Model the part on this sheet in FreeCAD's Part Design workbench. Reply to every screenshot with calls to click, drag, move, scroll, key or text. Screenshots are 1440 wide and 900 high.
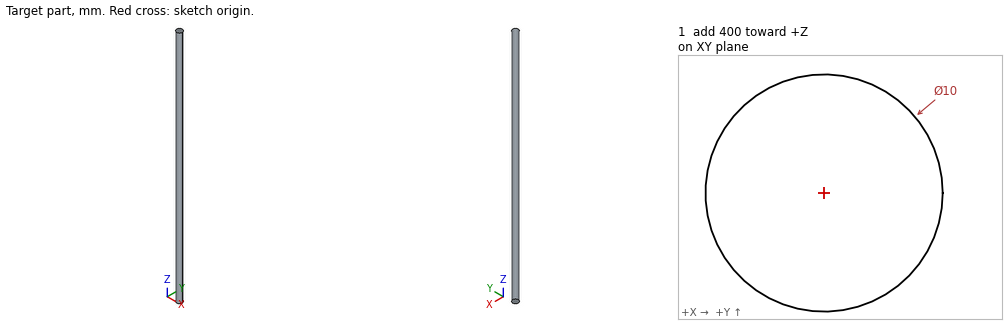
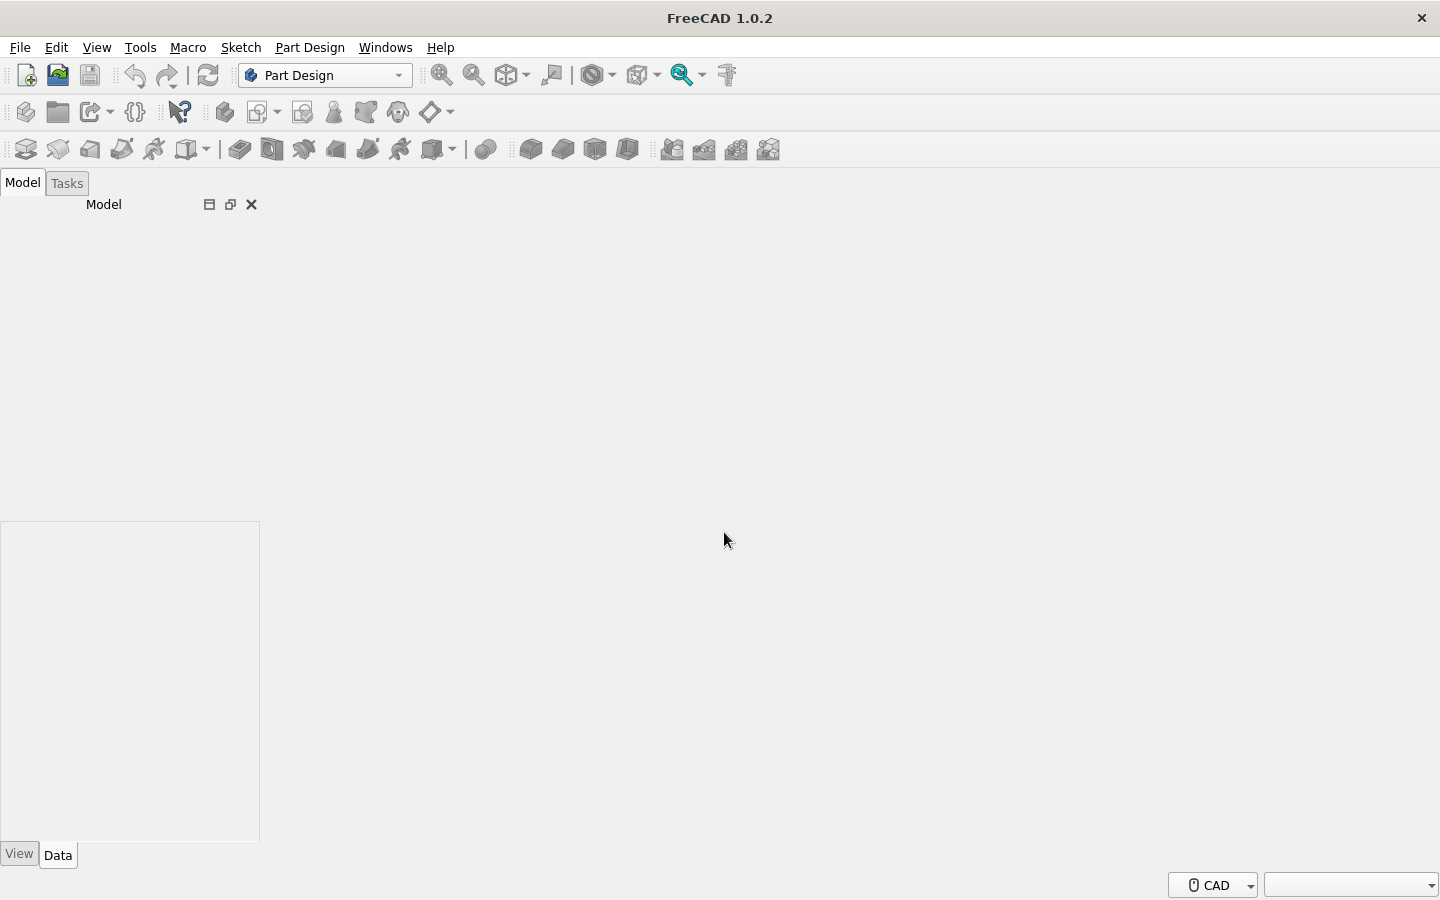
click(26, 76)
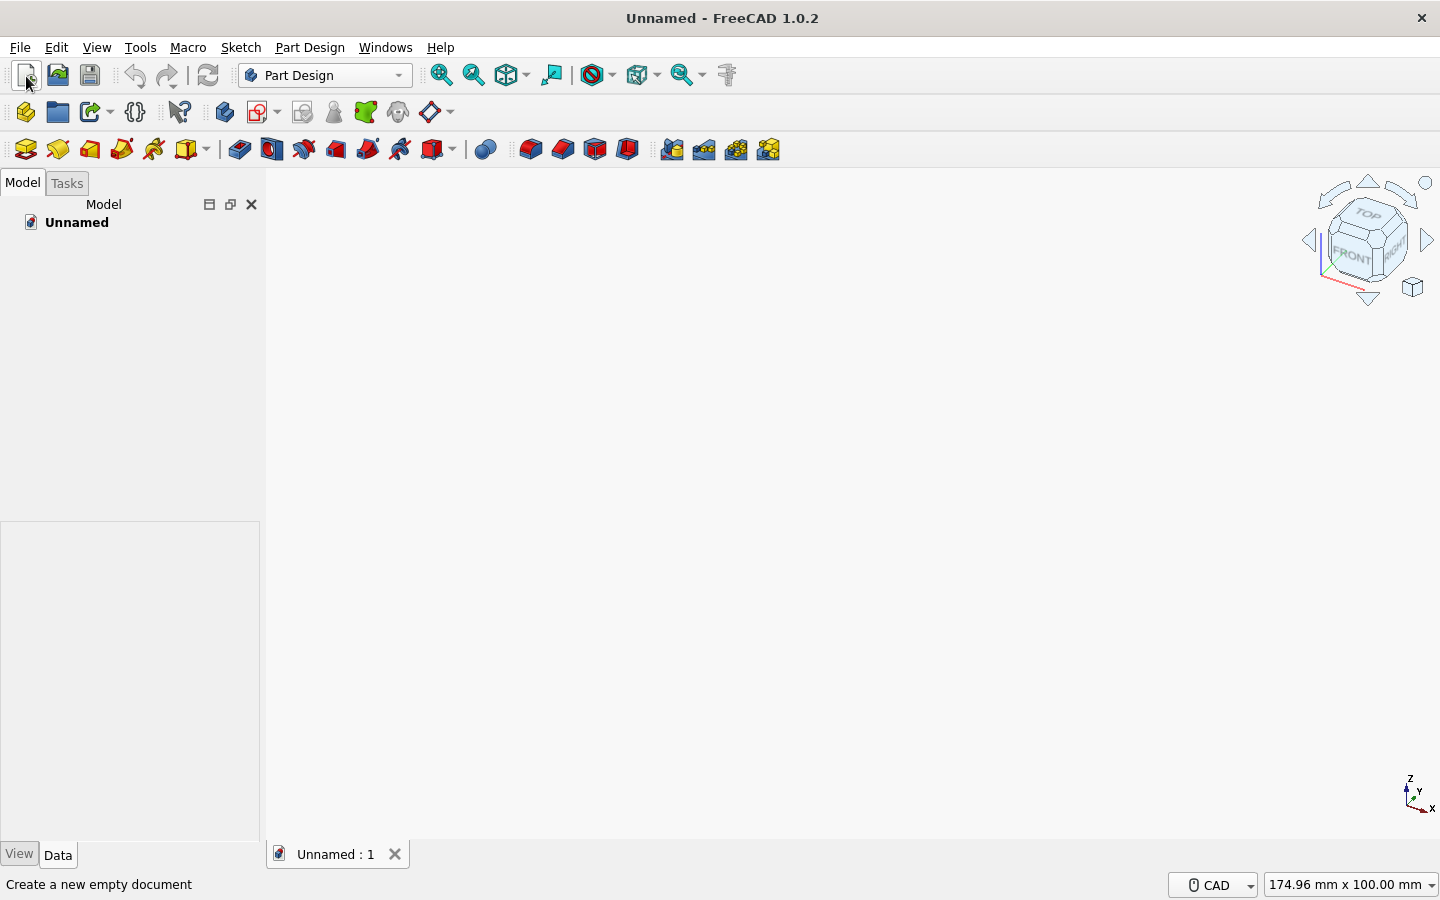
click(258, 112)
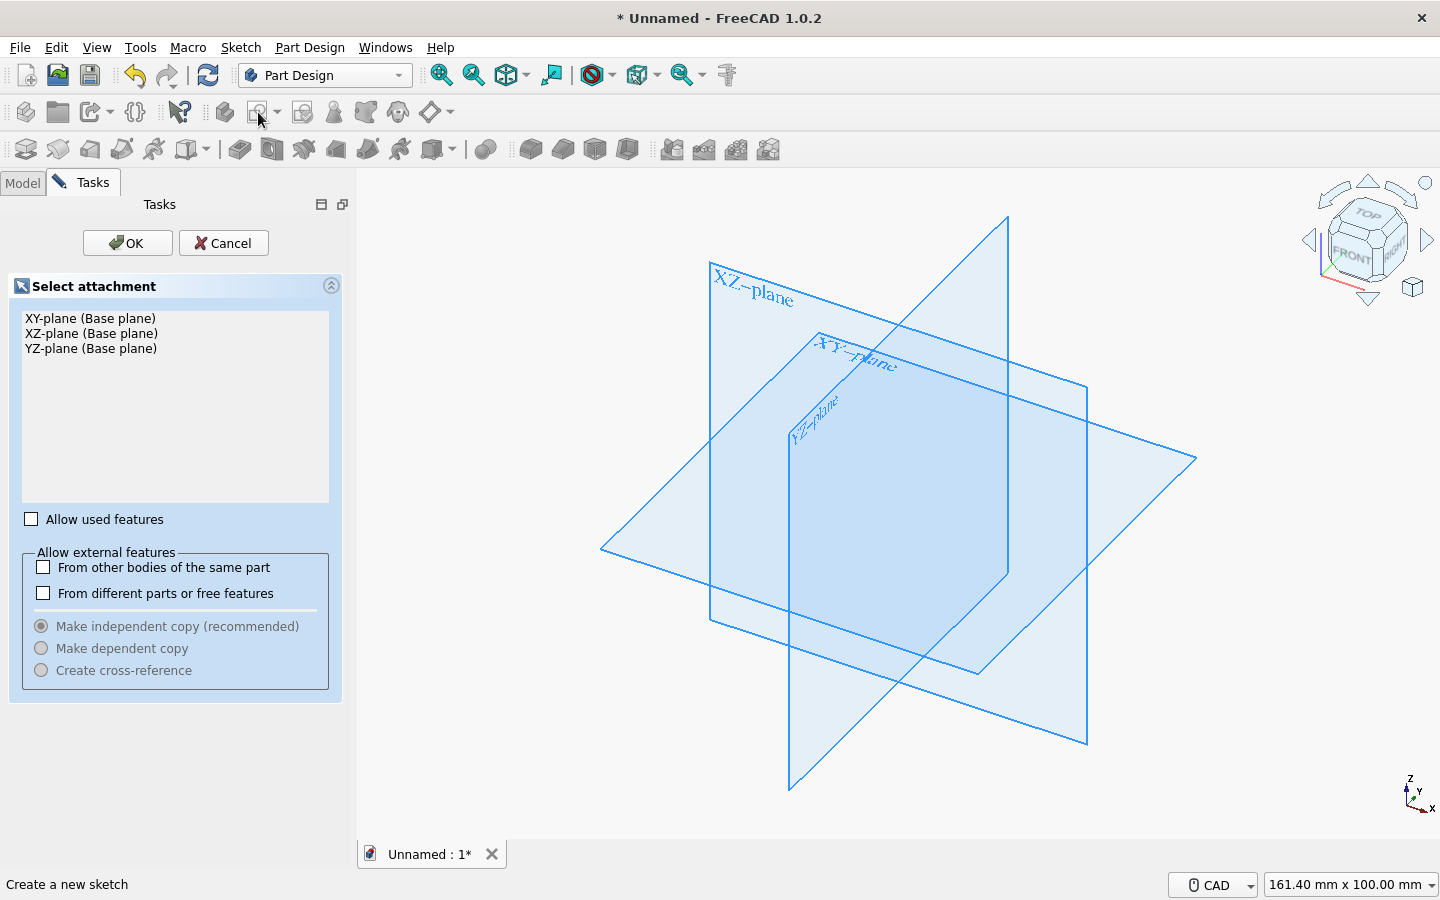
click(82, 318)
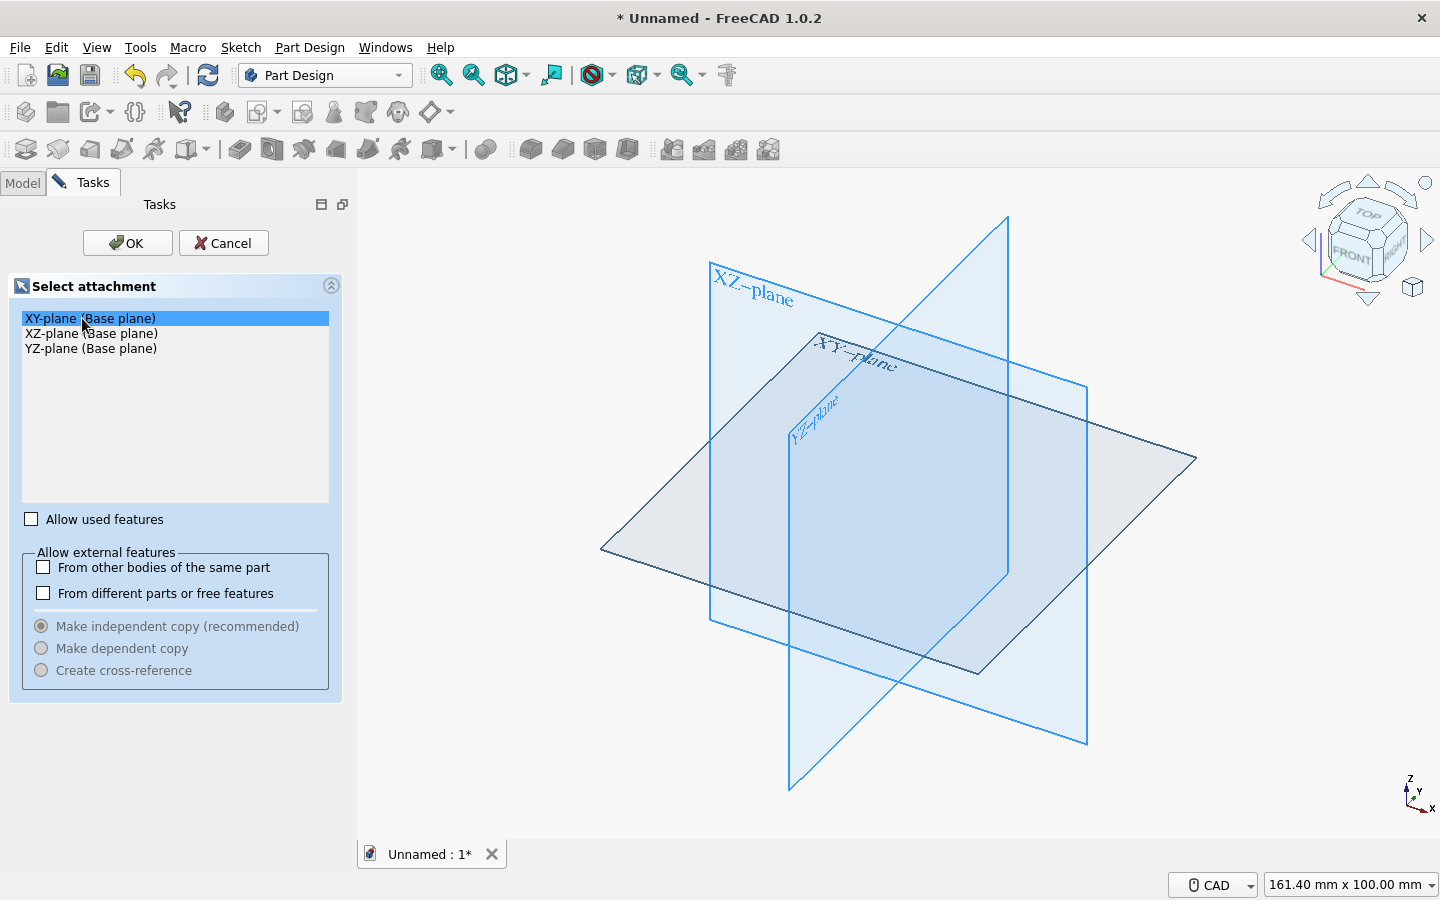
click(128, 243)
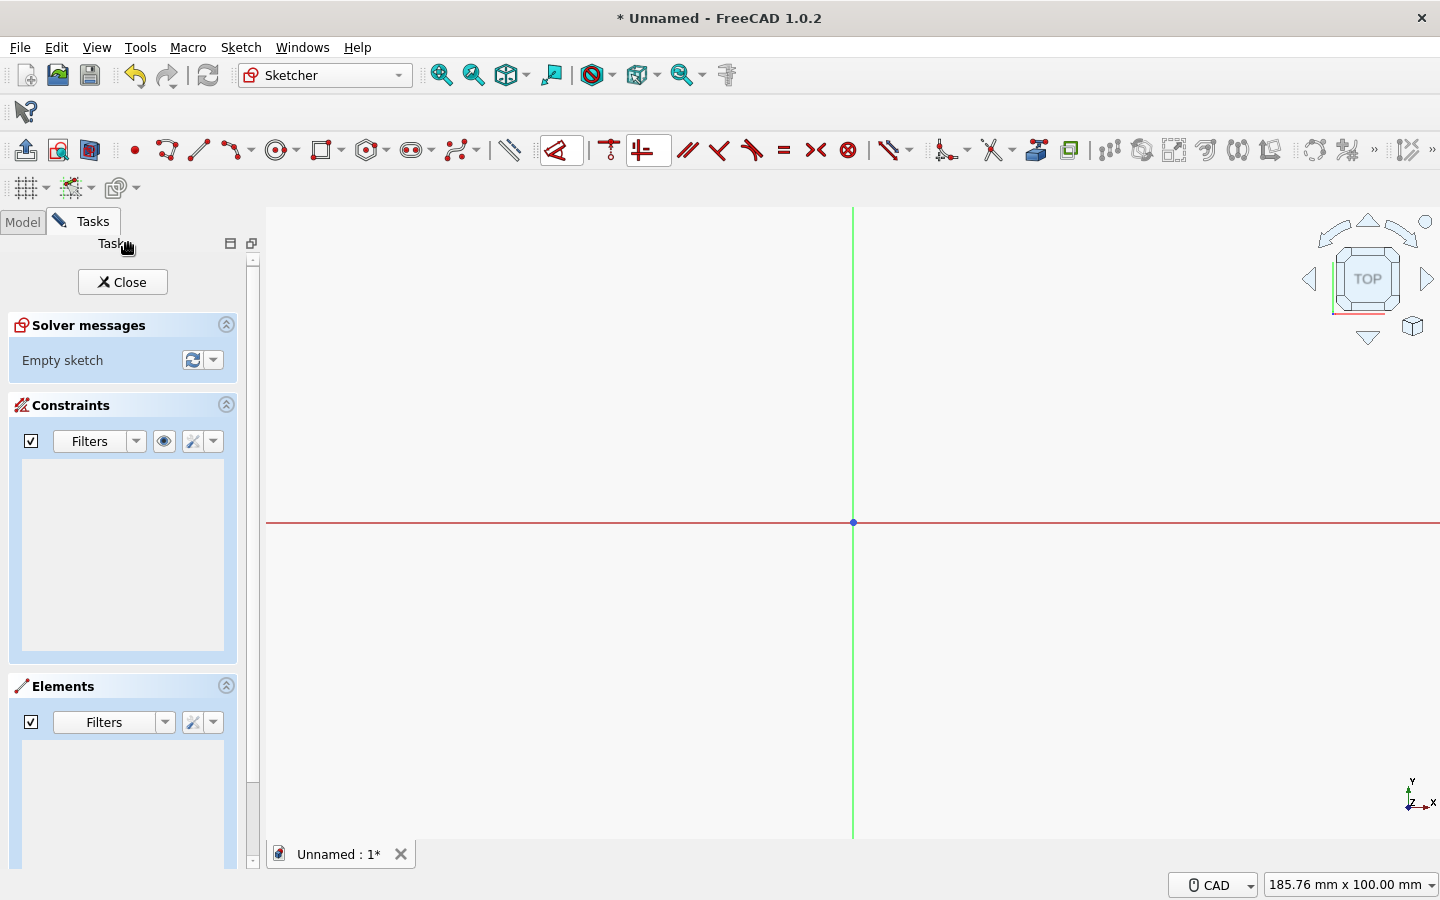
scroll(867, 523, up, 9)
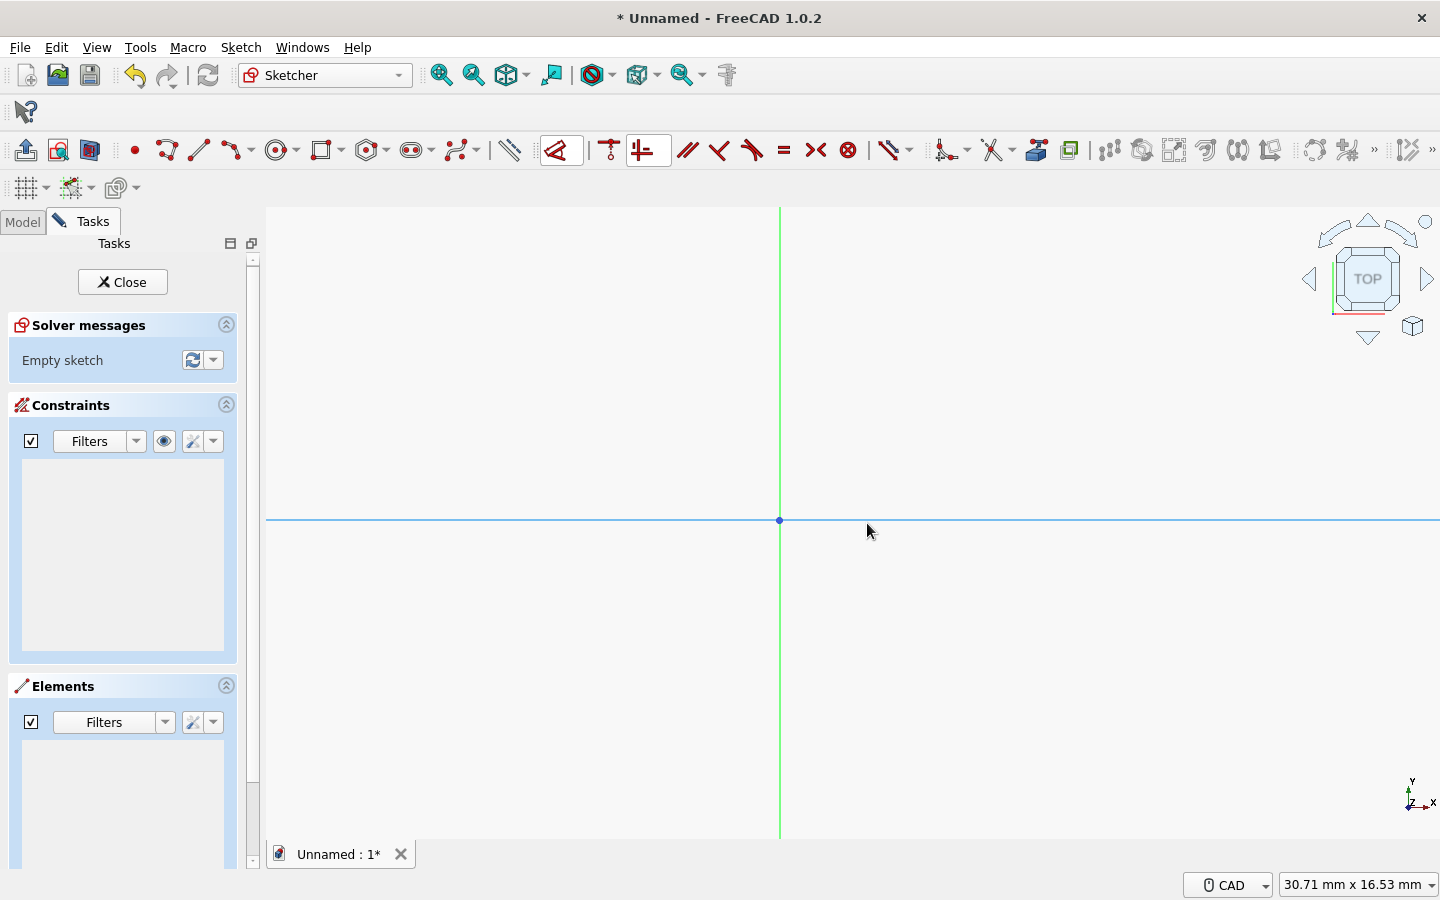
click(276, 150)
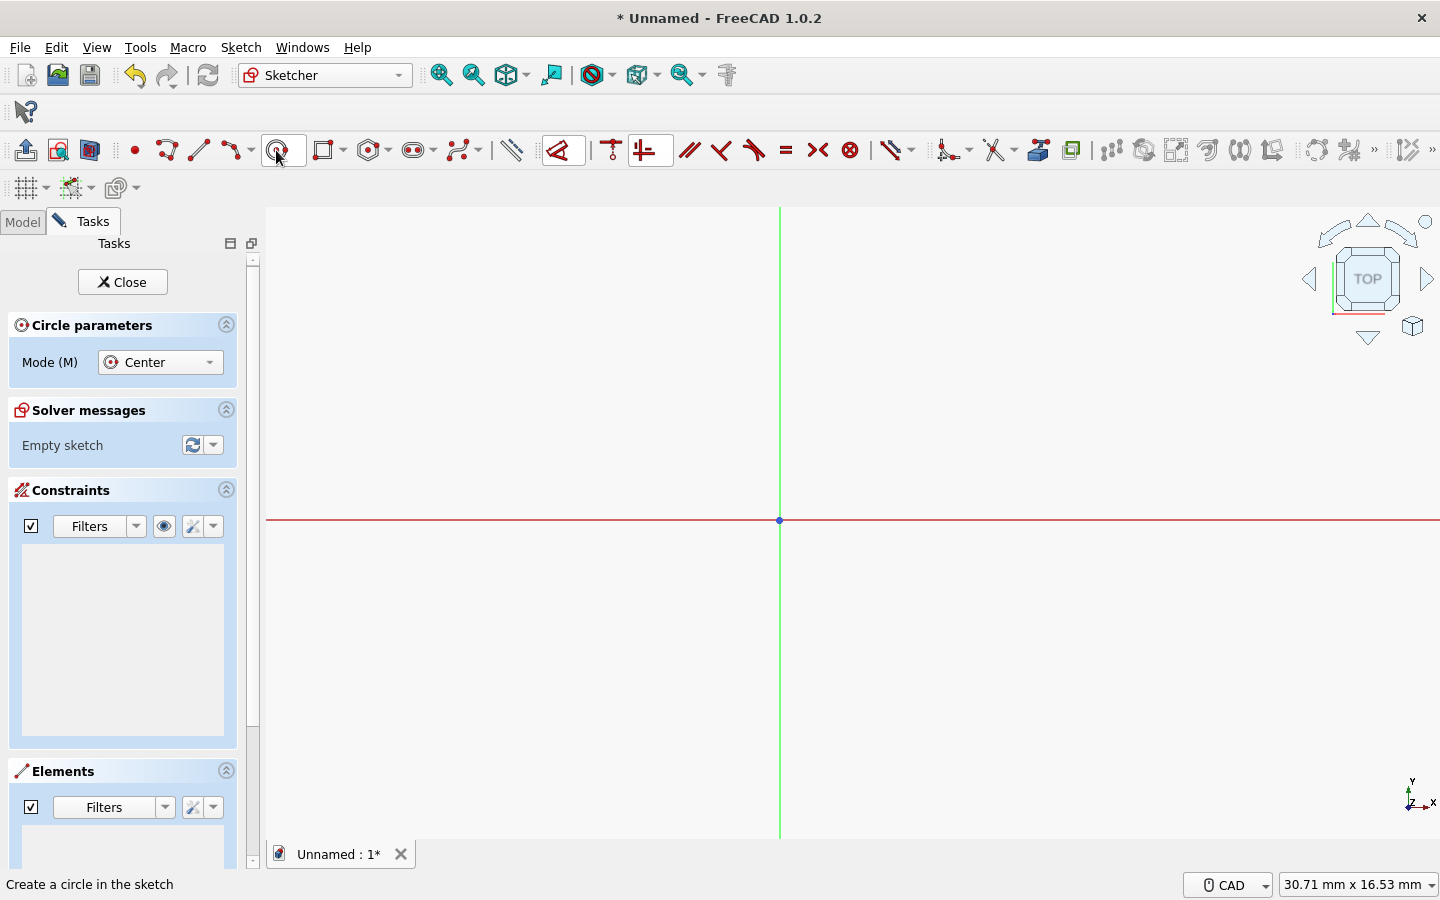
click(780, 520)
click(915, 385)
key(Escape)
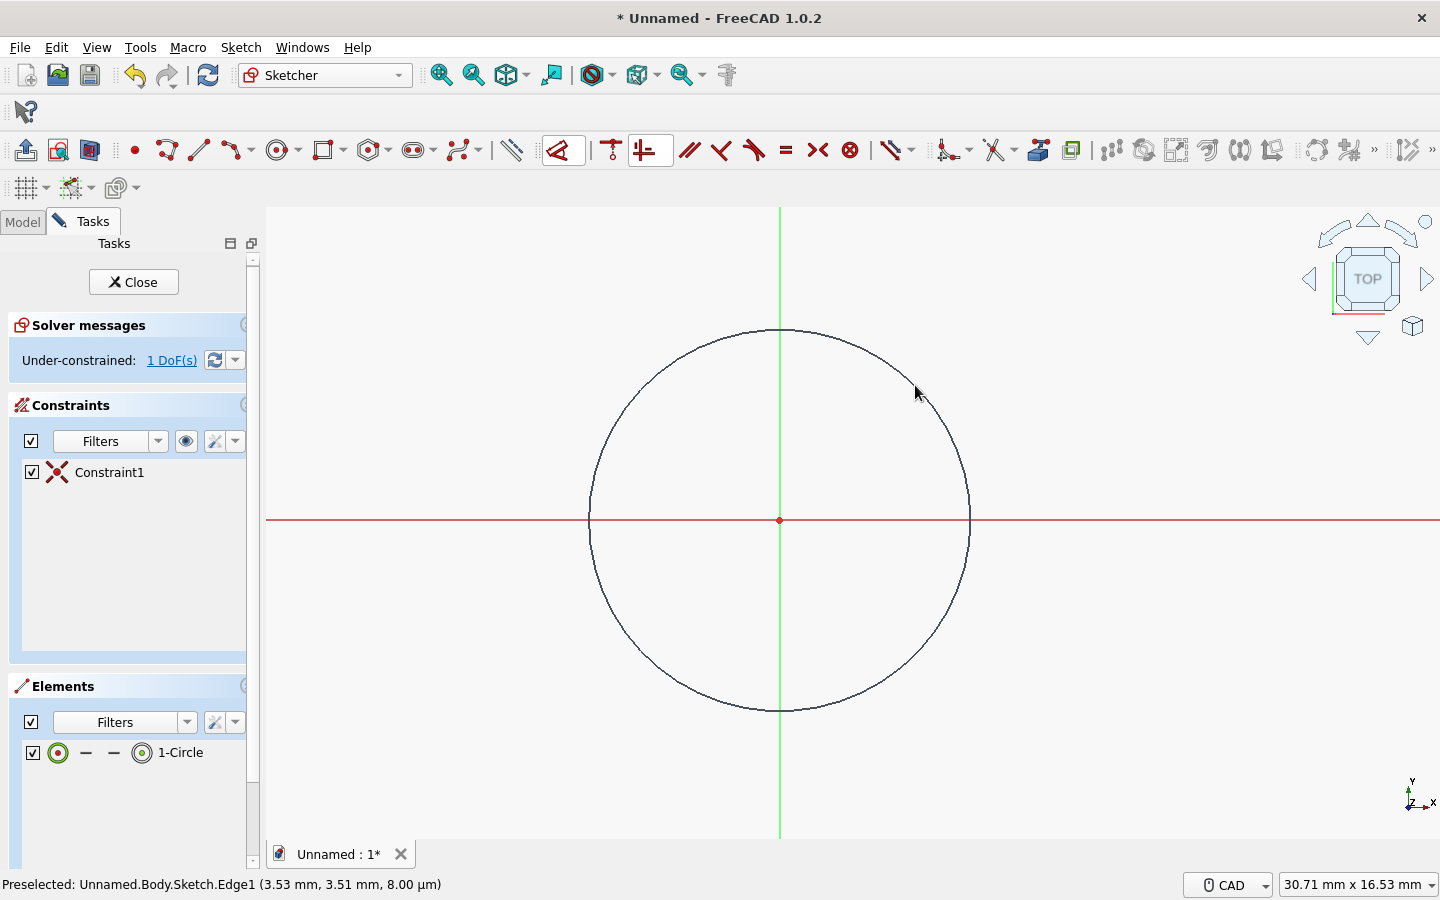
click(558, 150)